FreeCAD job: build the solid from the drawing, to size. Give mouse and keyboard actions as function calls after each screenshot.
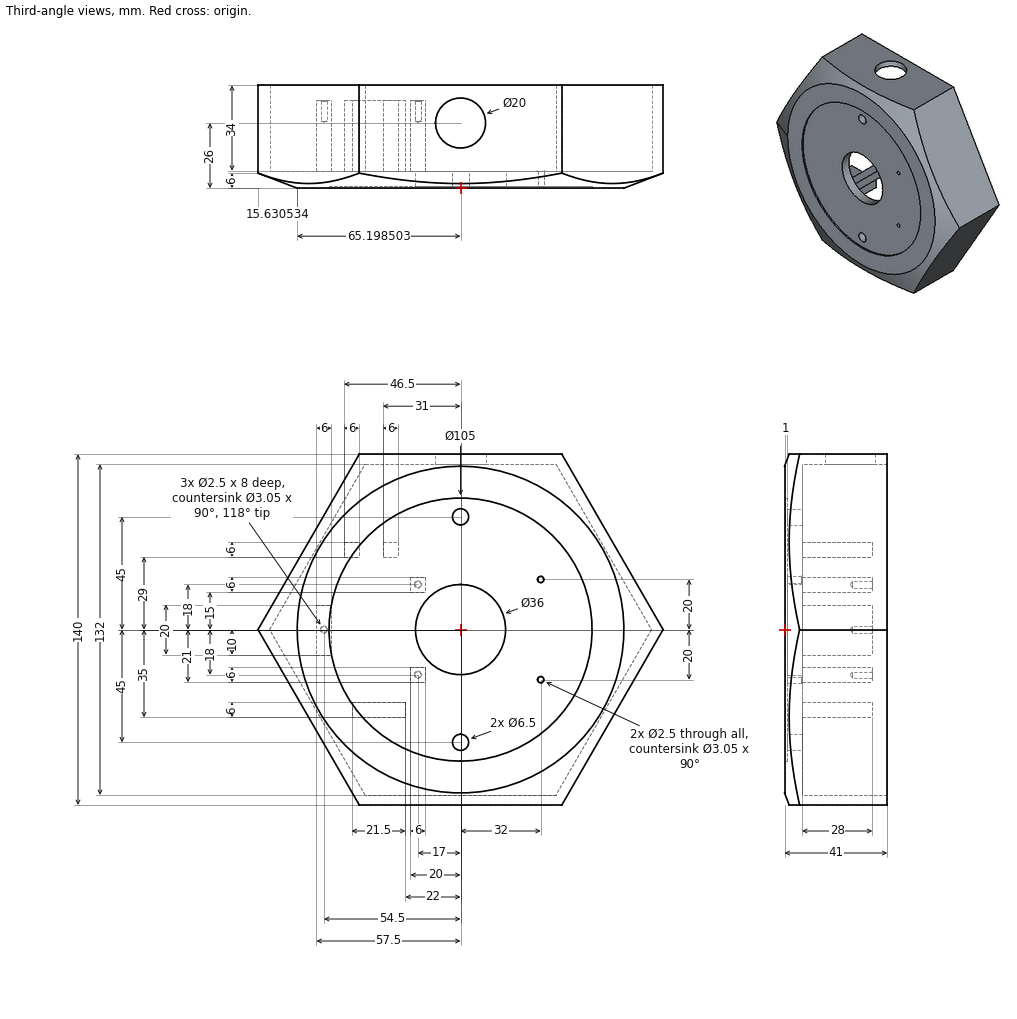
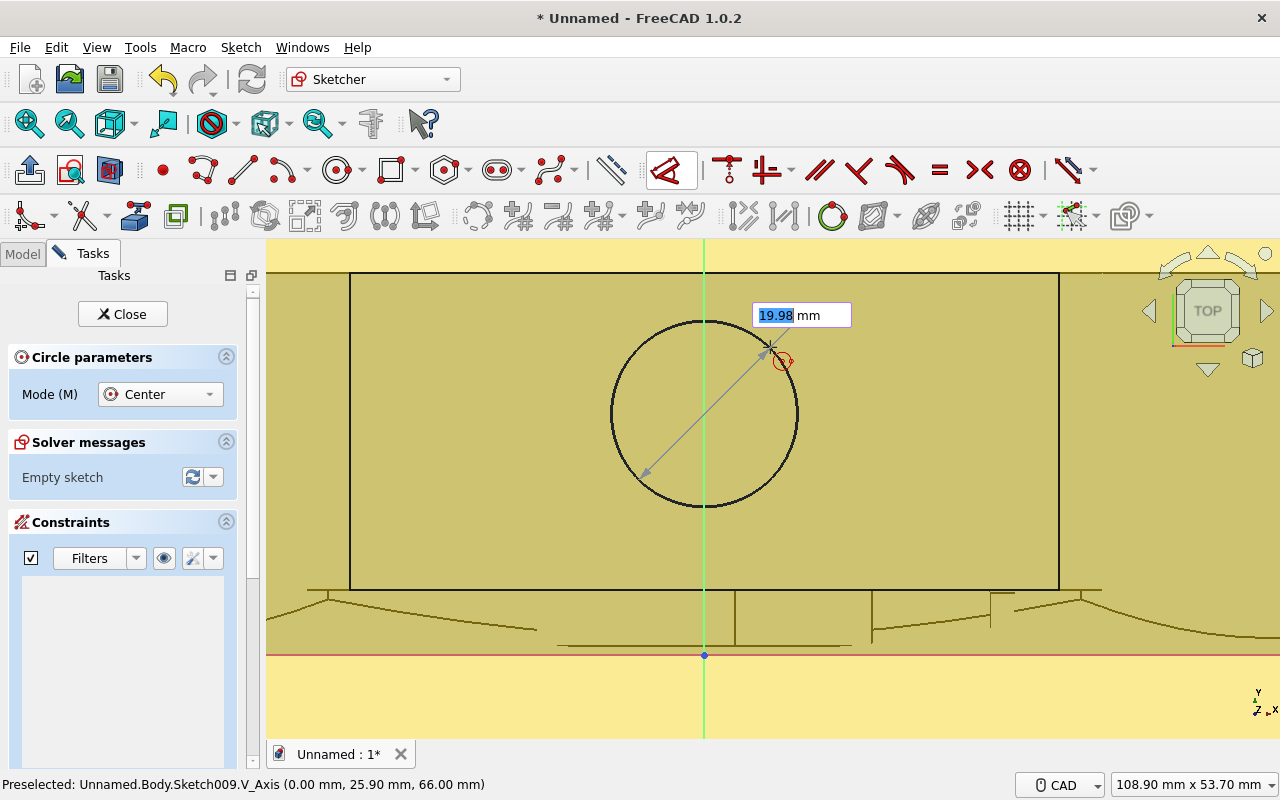
text(20)
key(Return)
key(Escape)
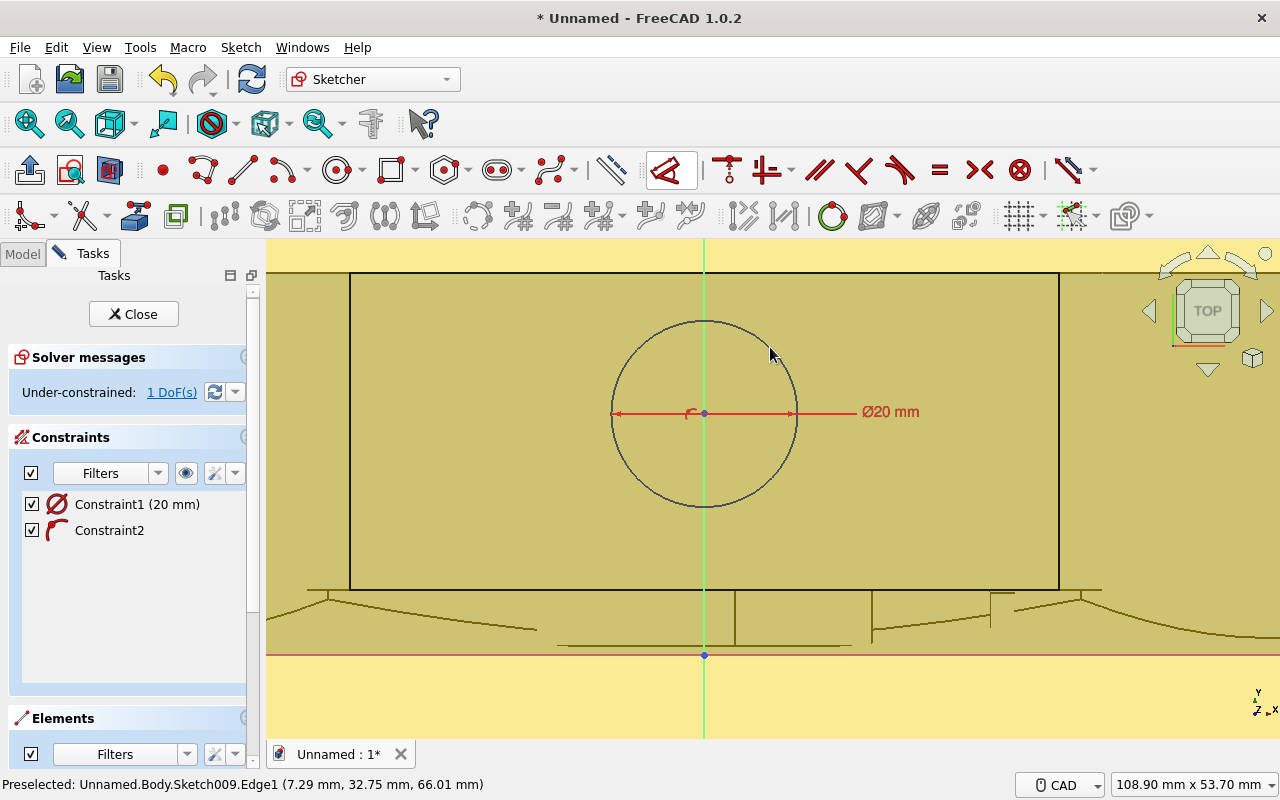
click(704, 414)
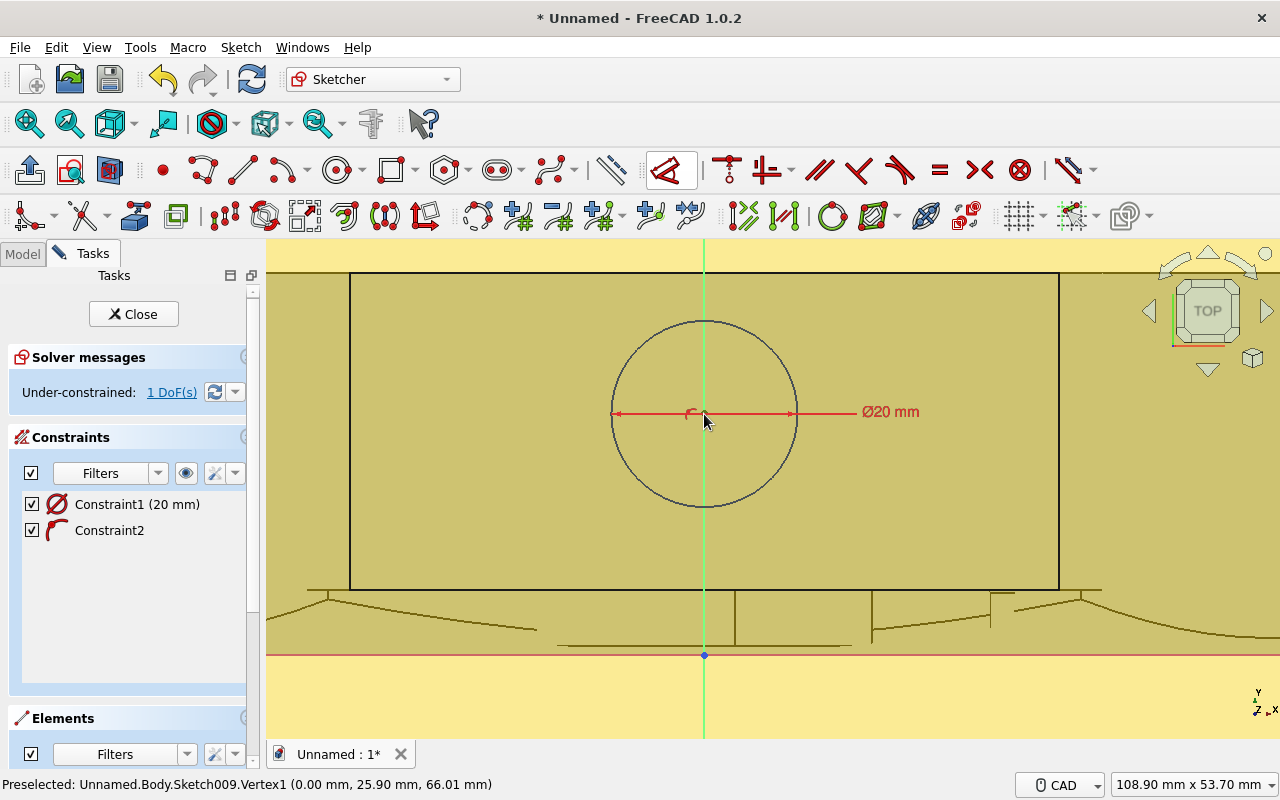
key(i)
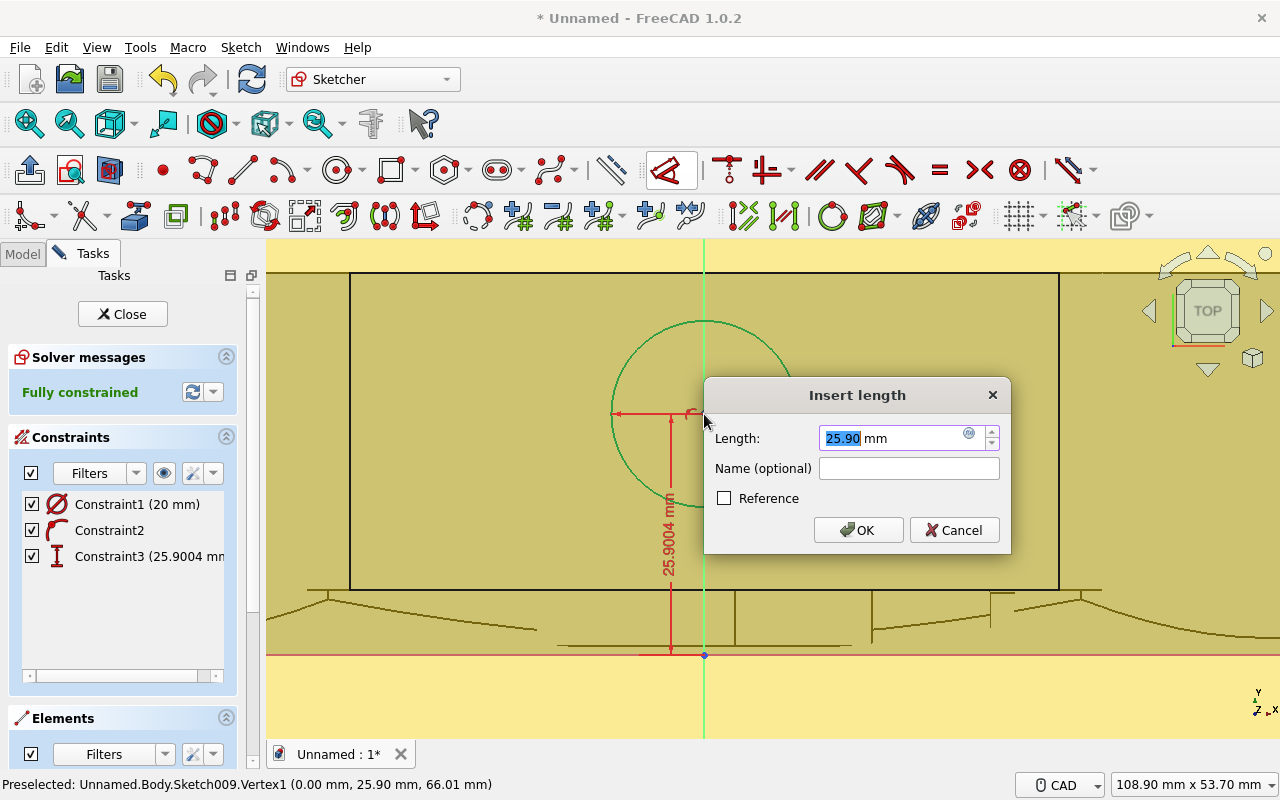
text(26)
key(Return)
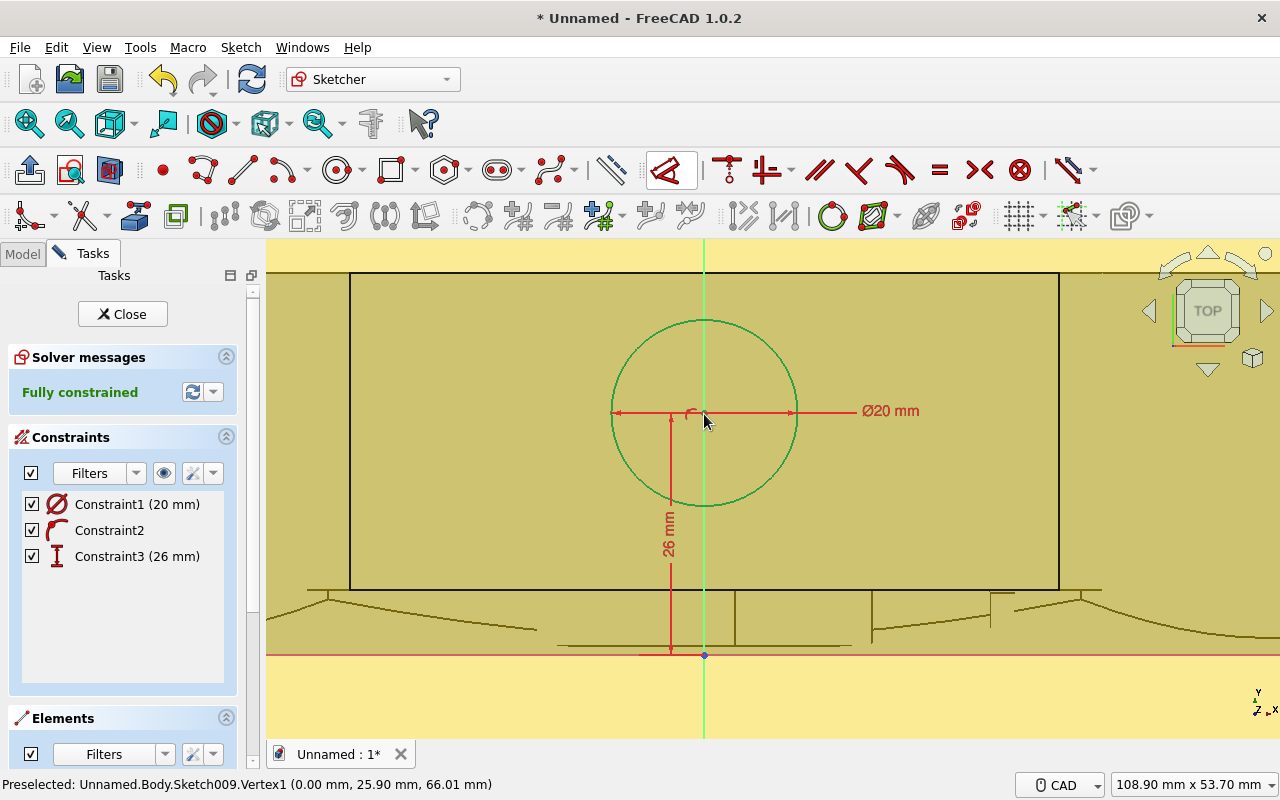
click(123, 314)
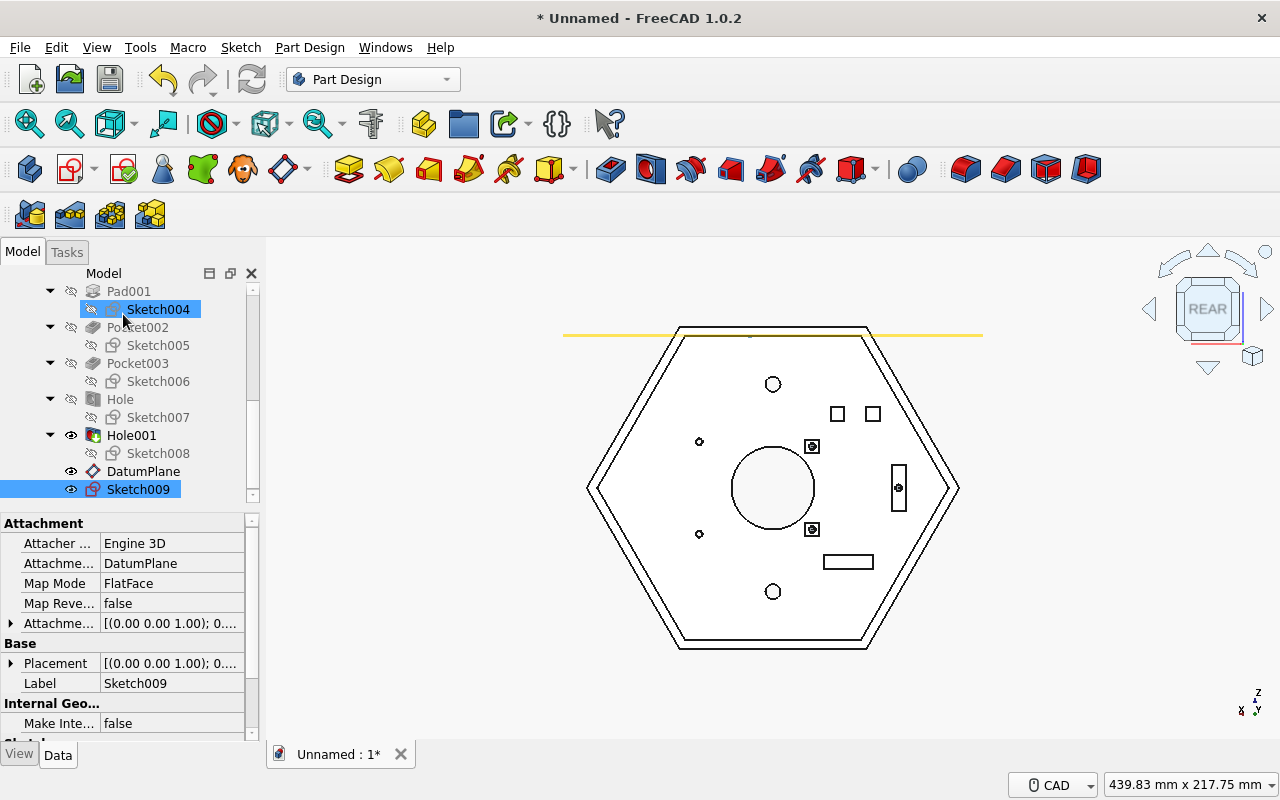
click(612, 170)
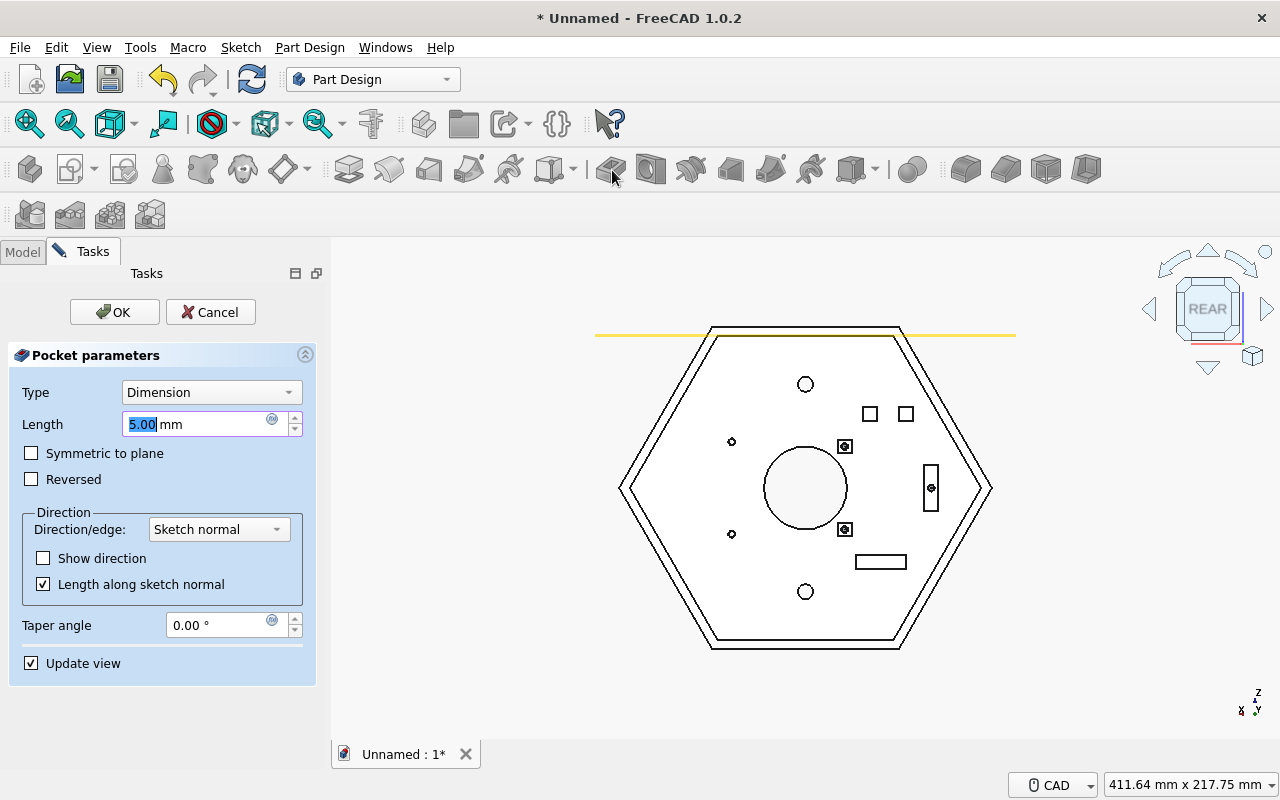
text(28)
key(Tab)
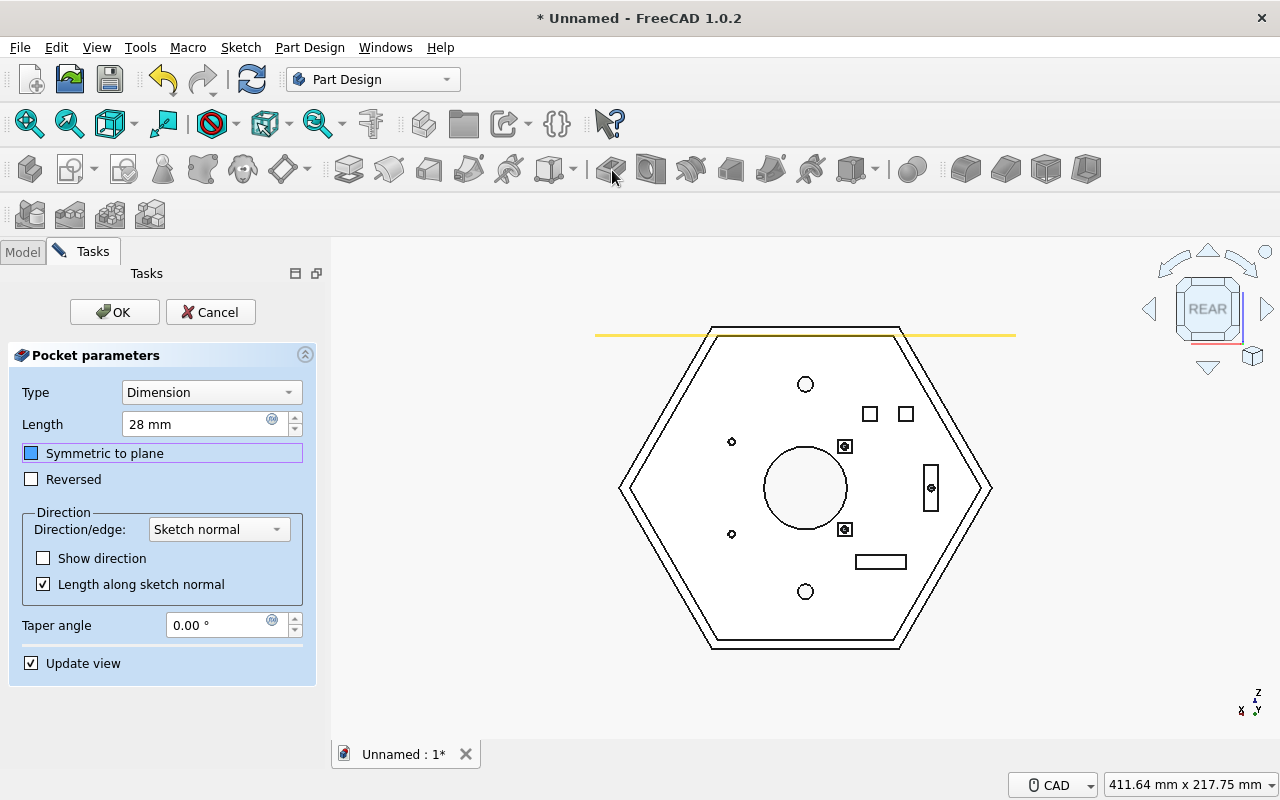
click(30, 479)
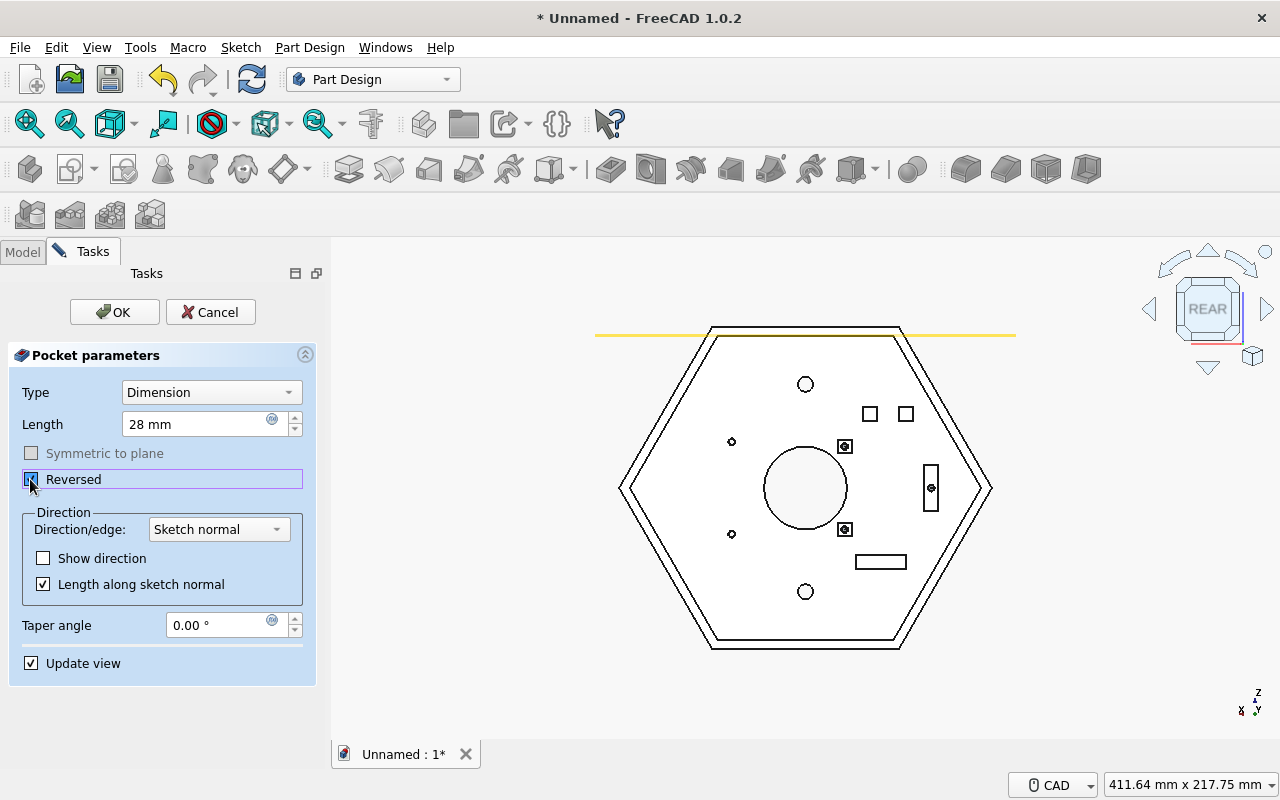
click(115, 312)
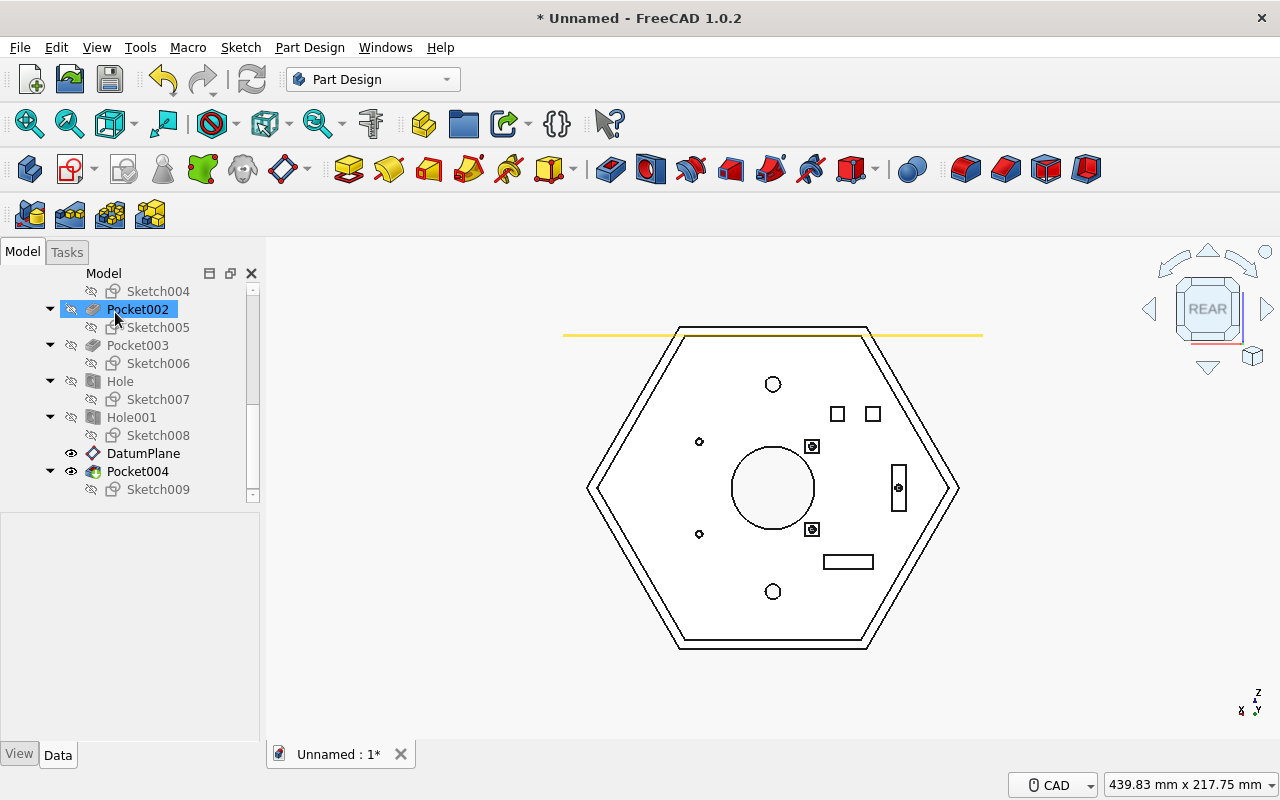
click(116, 453)
key(space)